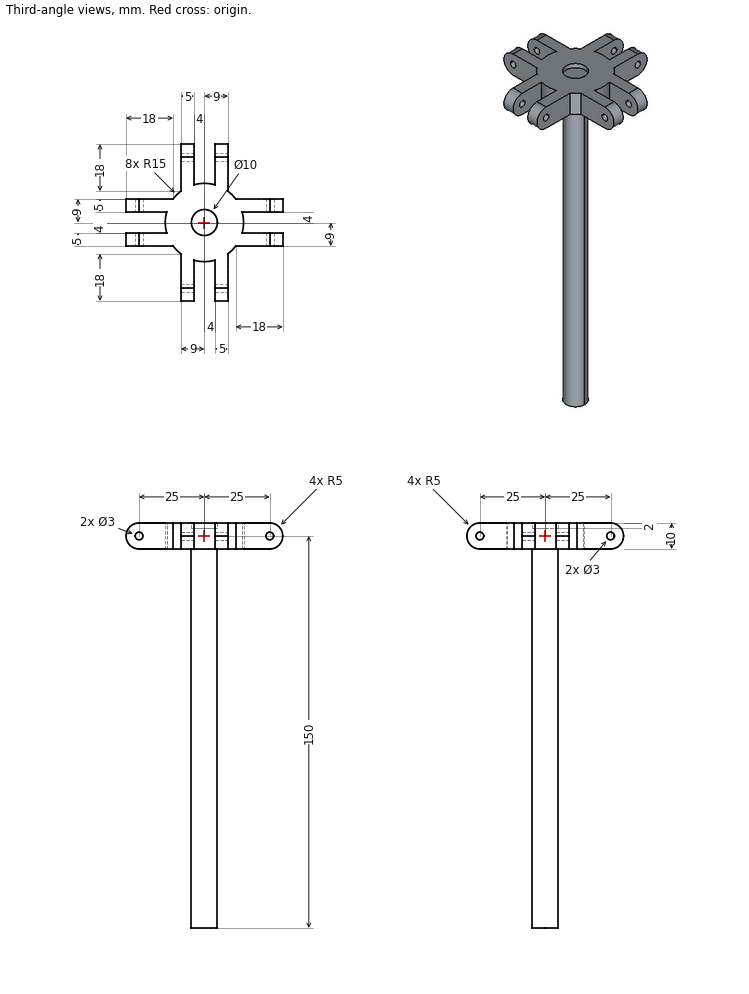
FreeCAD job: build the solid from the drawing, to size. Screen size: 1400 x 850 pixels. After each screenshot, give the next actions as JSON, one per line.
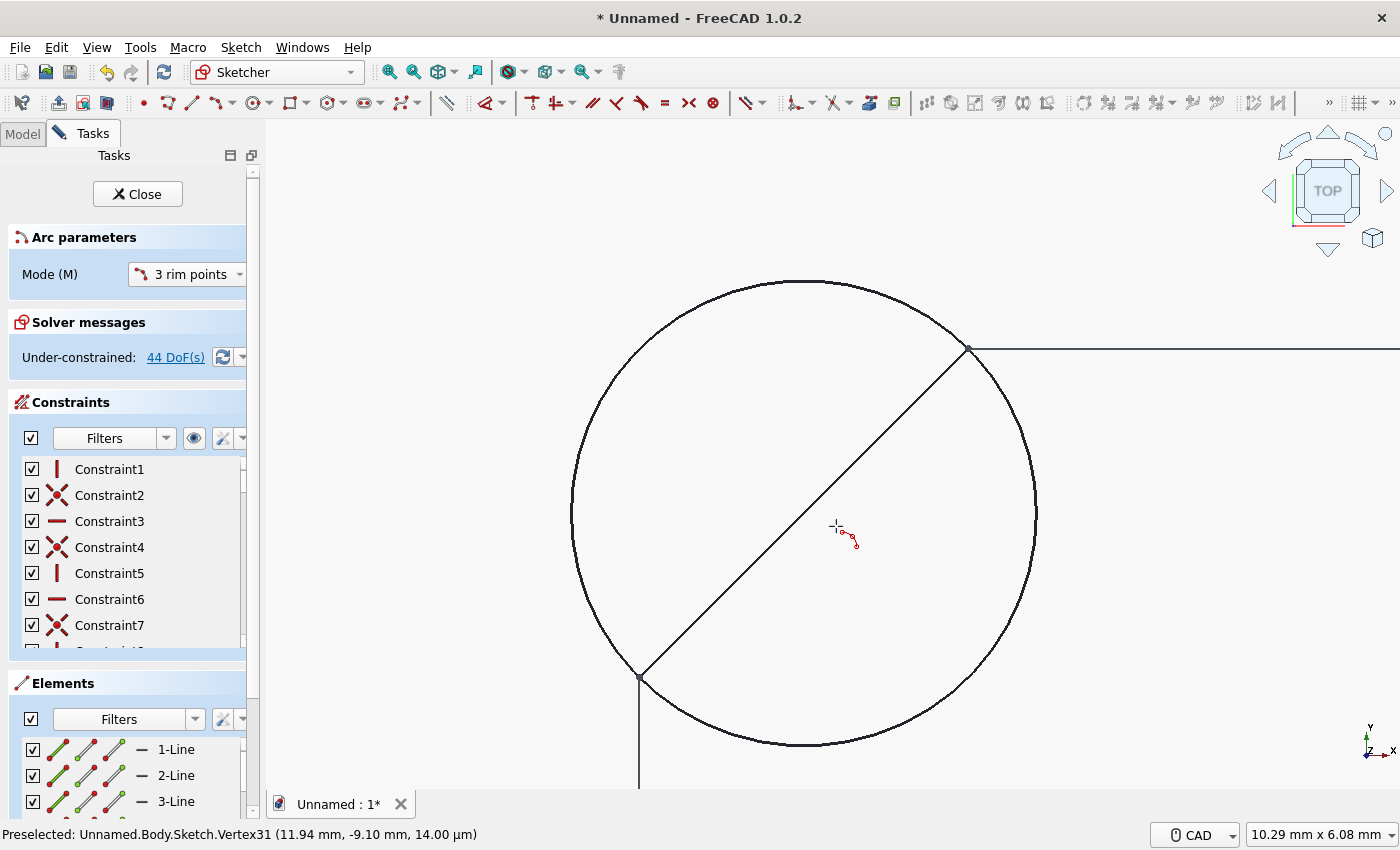
{"action": "left_click", "coordinate": [821, 514]}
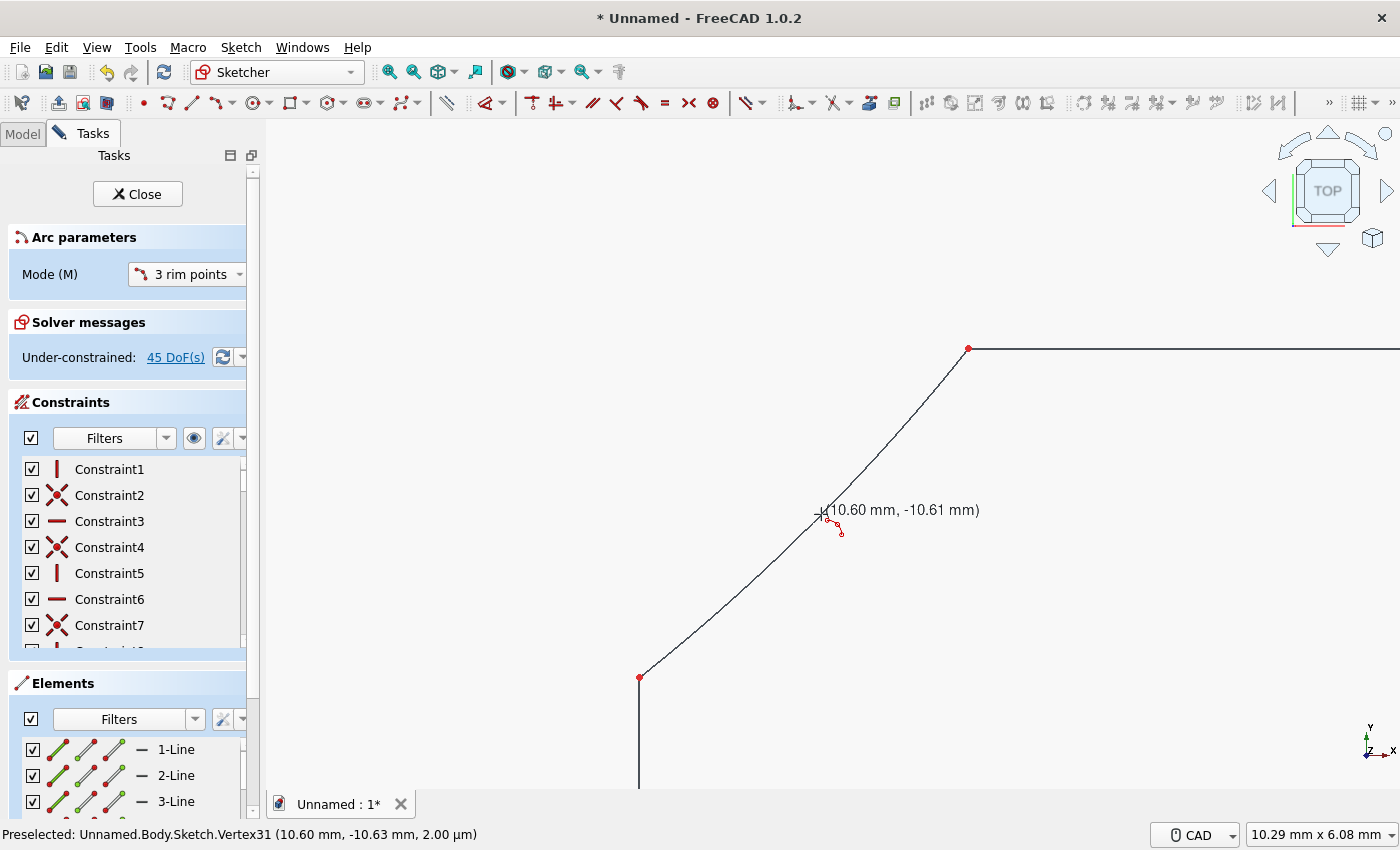
{"action": "scroll", "coordinate": [836, 526], "scroll_direction": "down", "scroll_amount": 14}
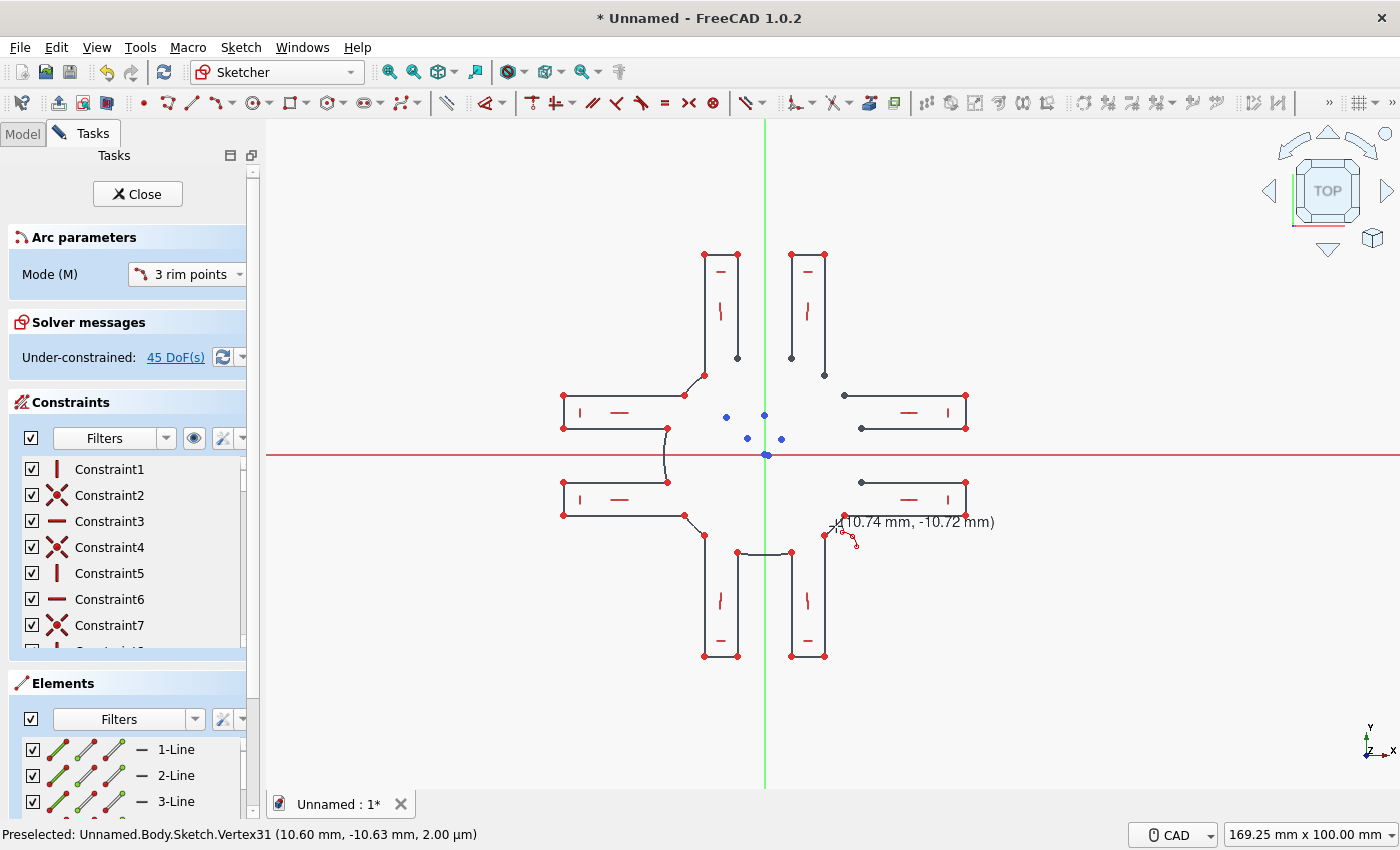
{"action": "left_click", "coordinate": [862, 483]}
{"action": "left_click", "coordinate": [862, 429]}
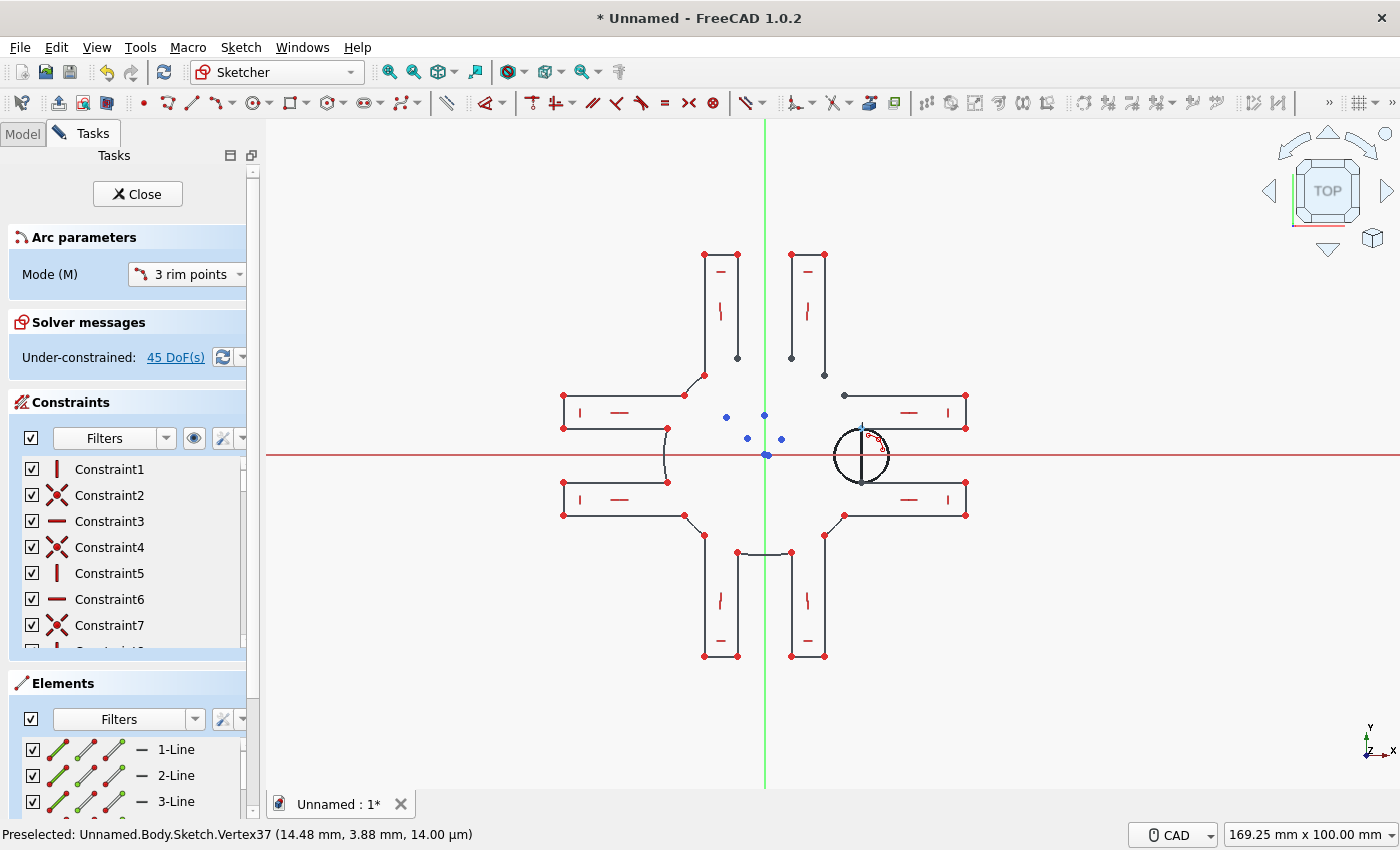
{"action": "scroll", "coordinate": [865, 460], "scroll_direction": "up", "scroll_amount": 8}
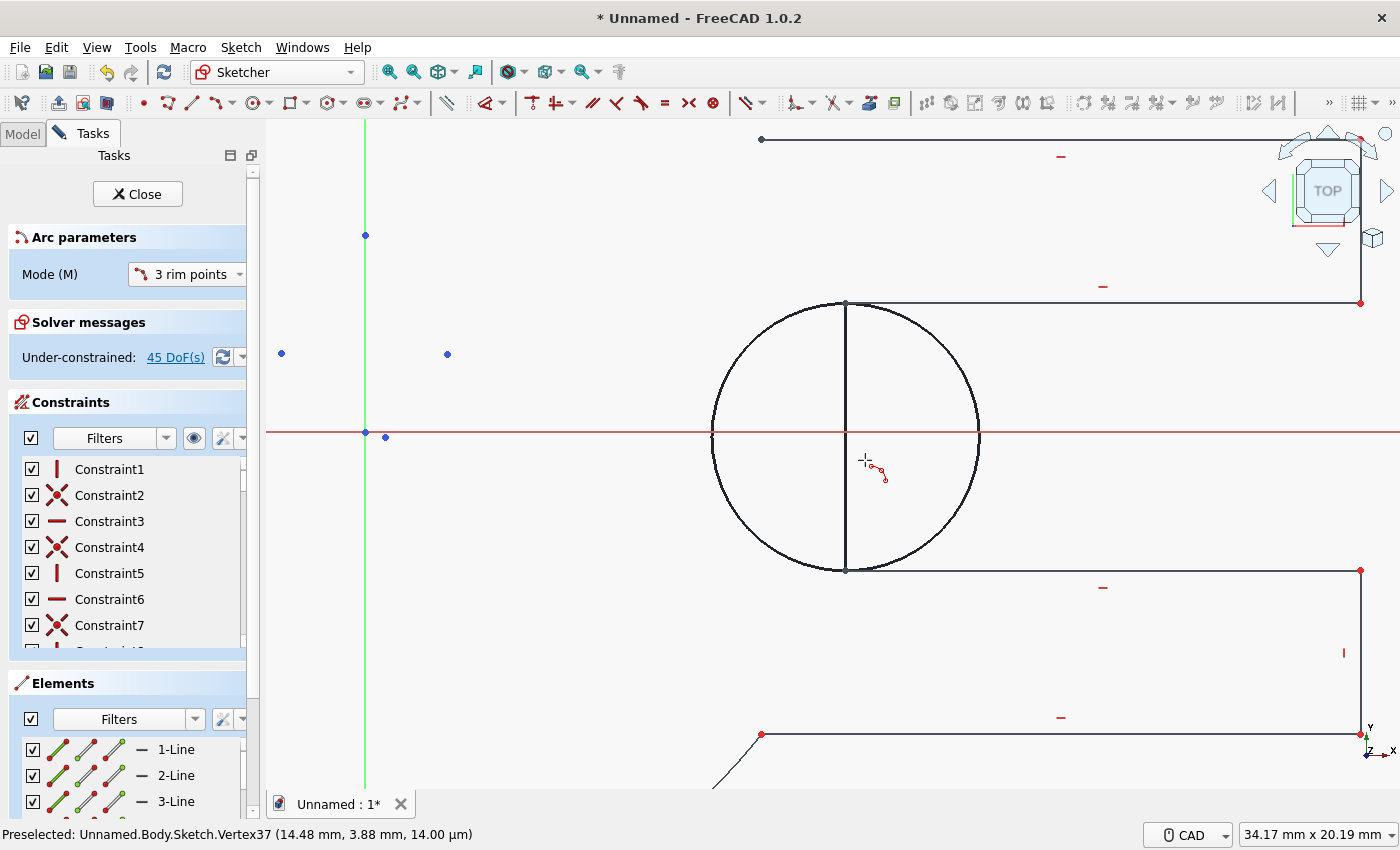
{"action": "left_click", "coordinate": [862, 459]}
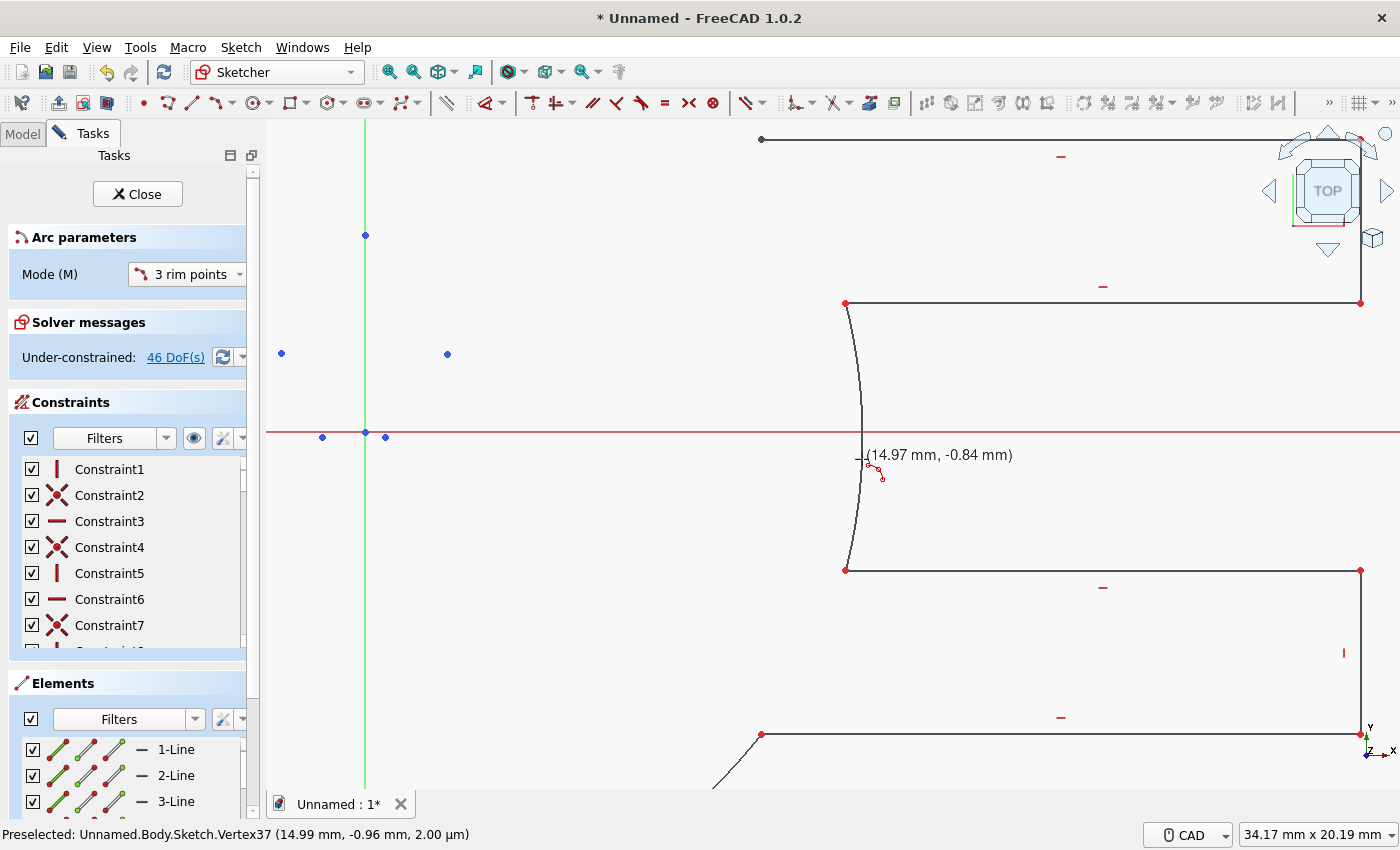
{"action": "scroll", "coordinate": [866, 460], "scroll_direction": "down", "scroll_amount": 8}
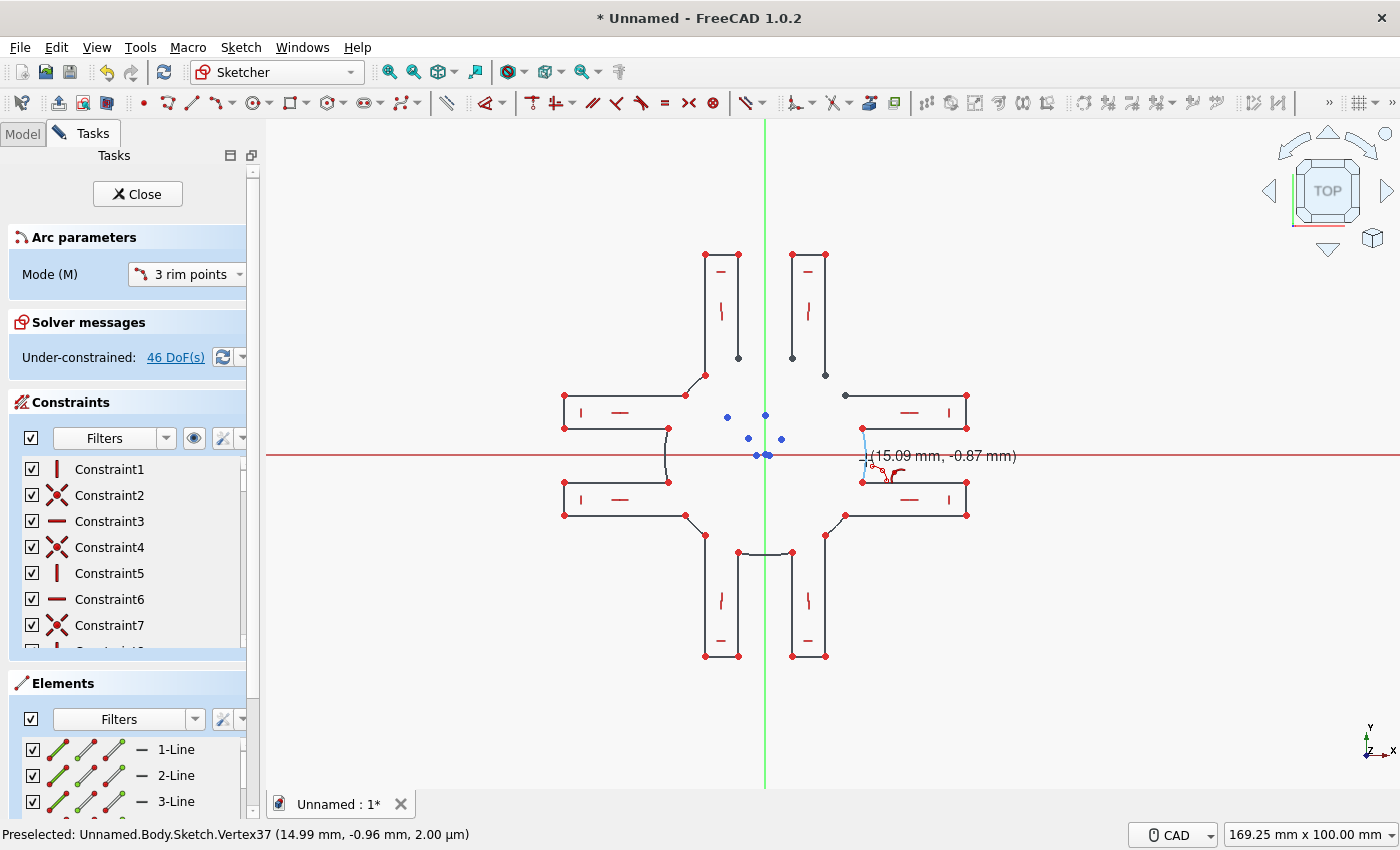
{"action": "left_click", "coordinate": [845, 396]}
{"action": "left_click", "coordinate": [825, 376]}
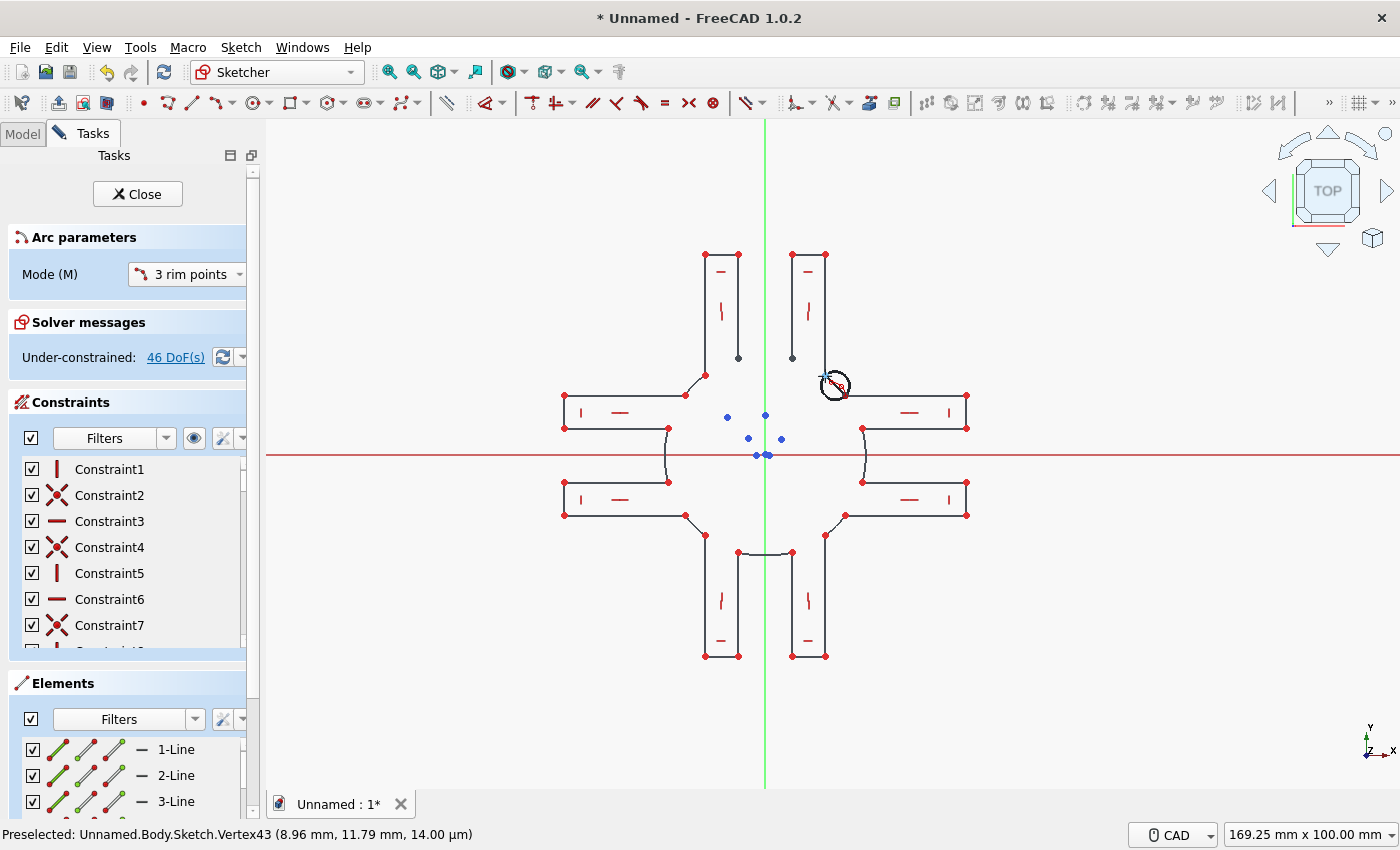
{"action": "scroll", "coordinate": [836, 384], "scroll_direction": "up", "scroll_amount": 14}